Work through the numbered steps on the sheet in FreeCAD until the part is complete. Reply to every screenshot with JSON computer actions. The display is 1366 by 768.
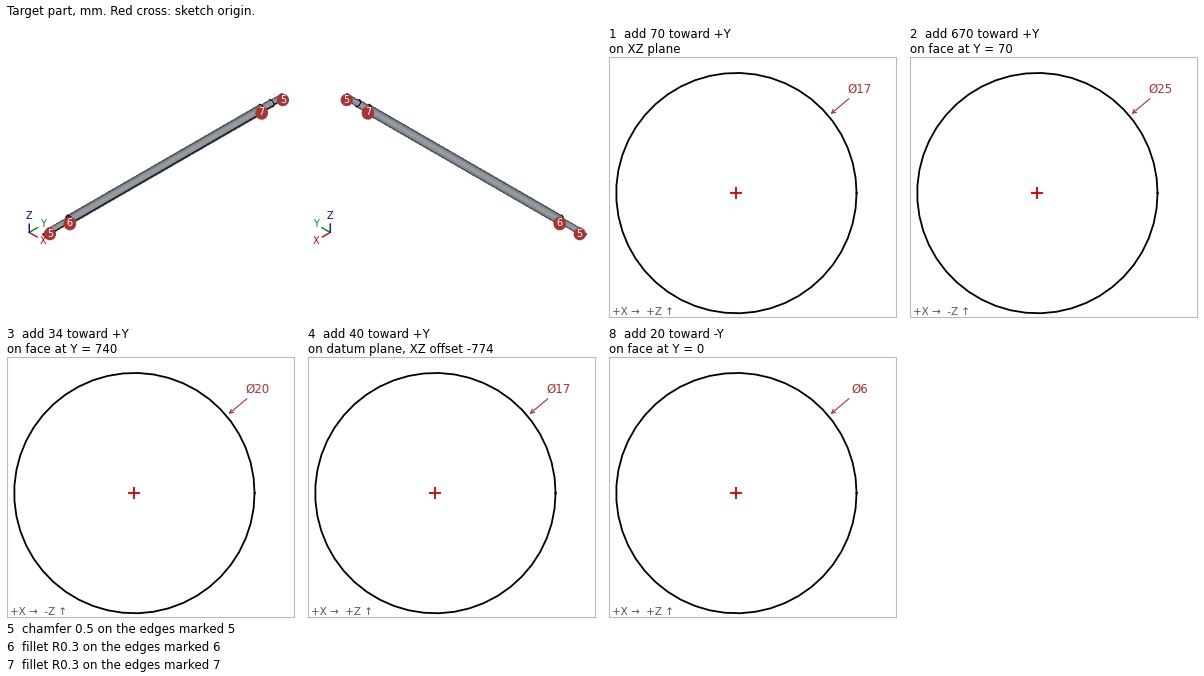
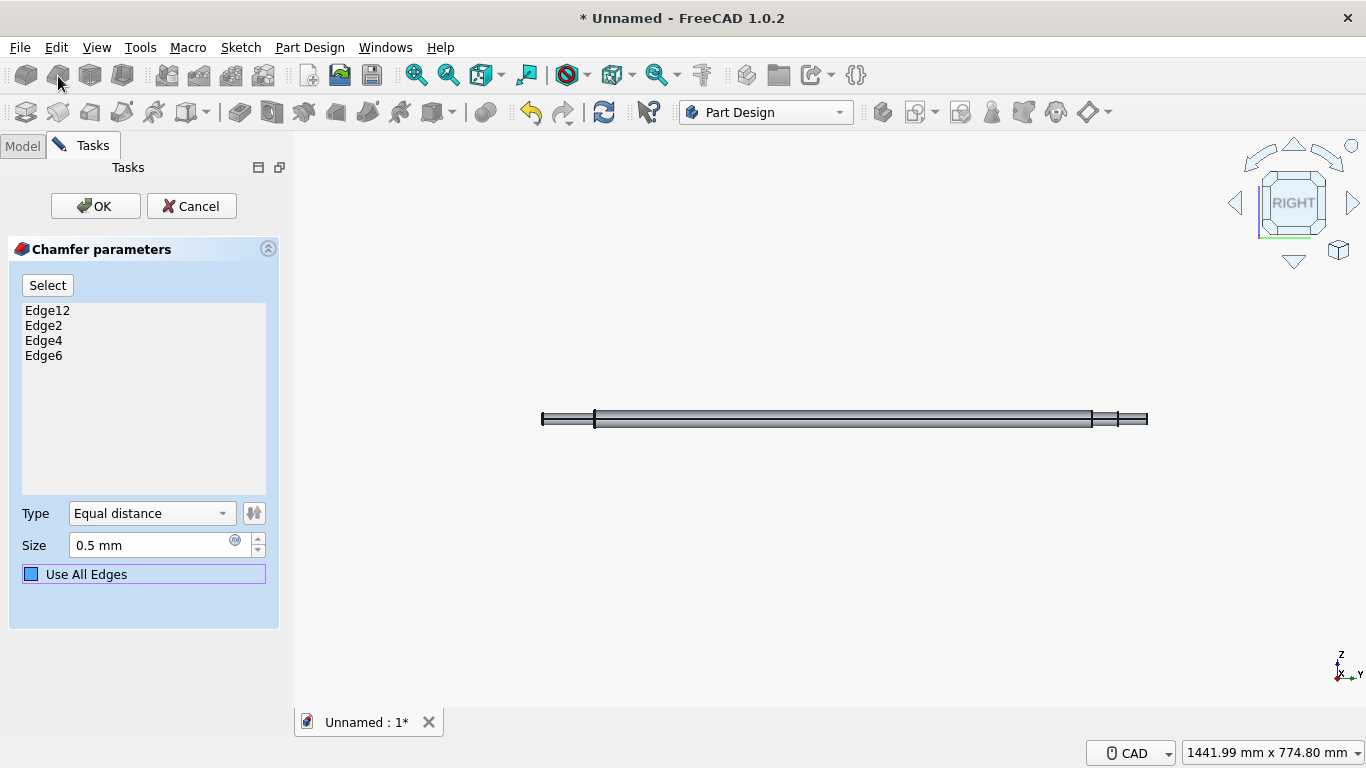
{"action": "left_click", "coordinate": [96, 206]}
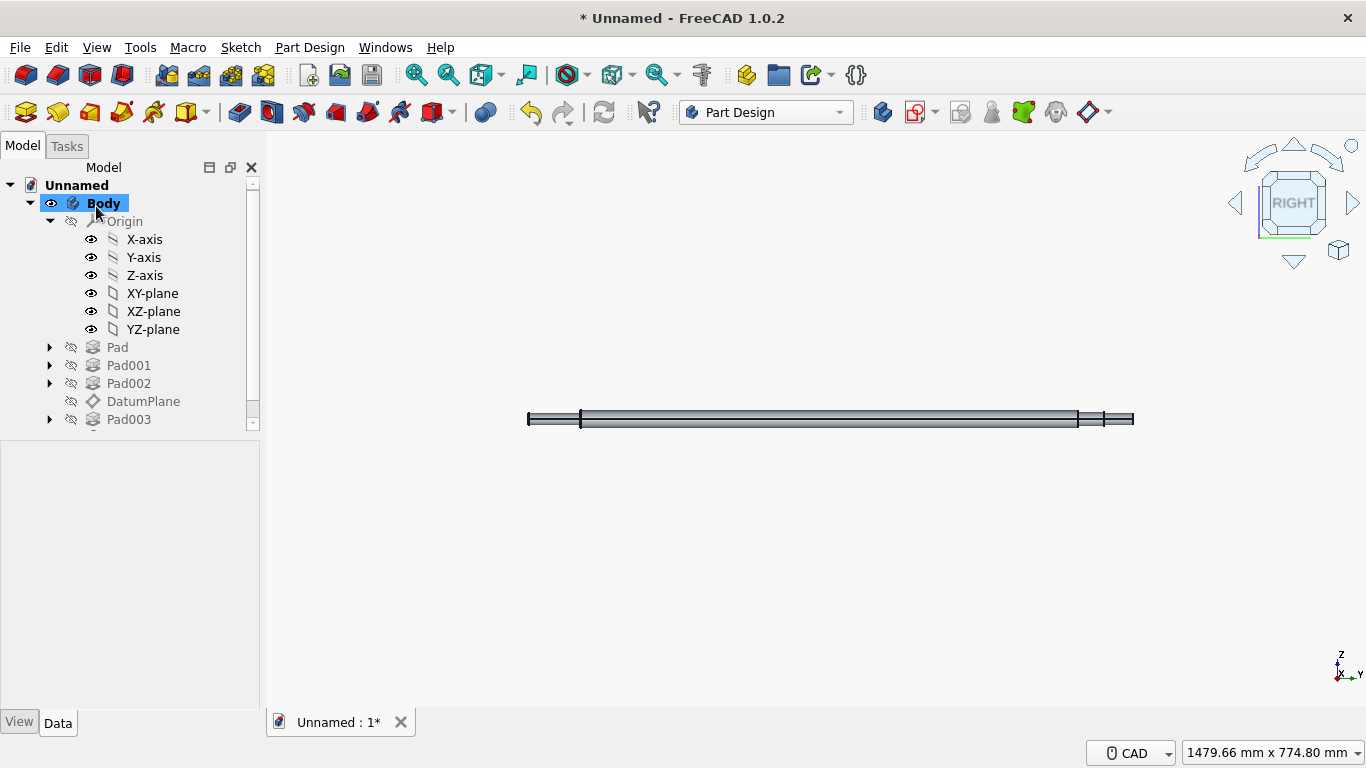
{"action": "key", "text": "0"}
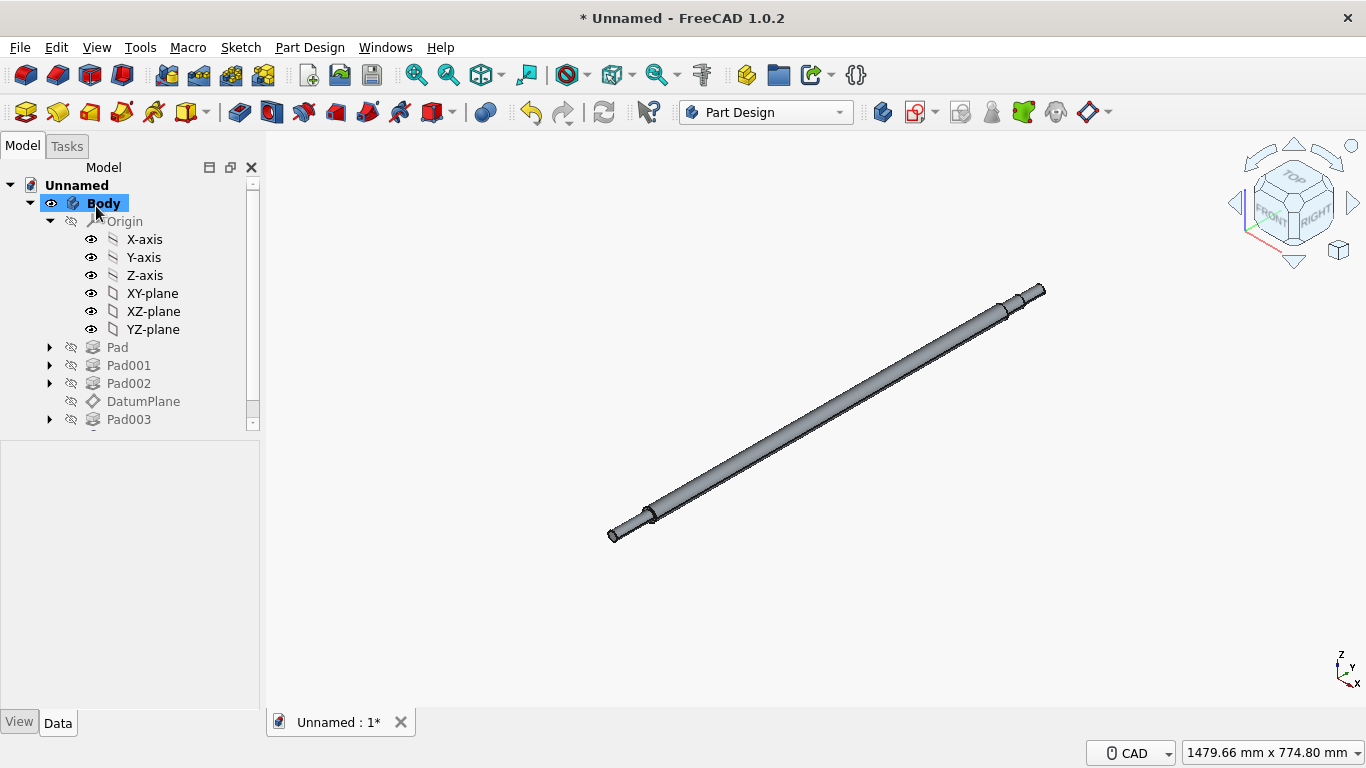
{"action": "key", "text": "2"}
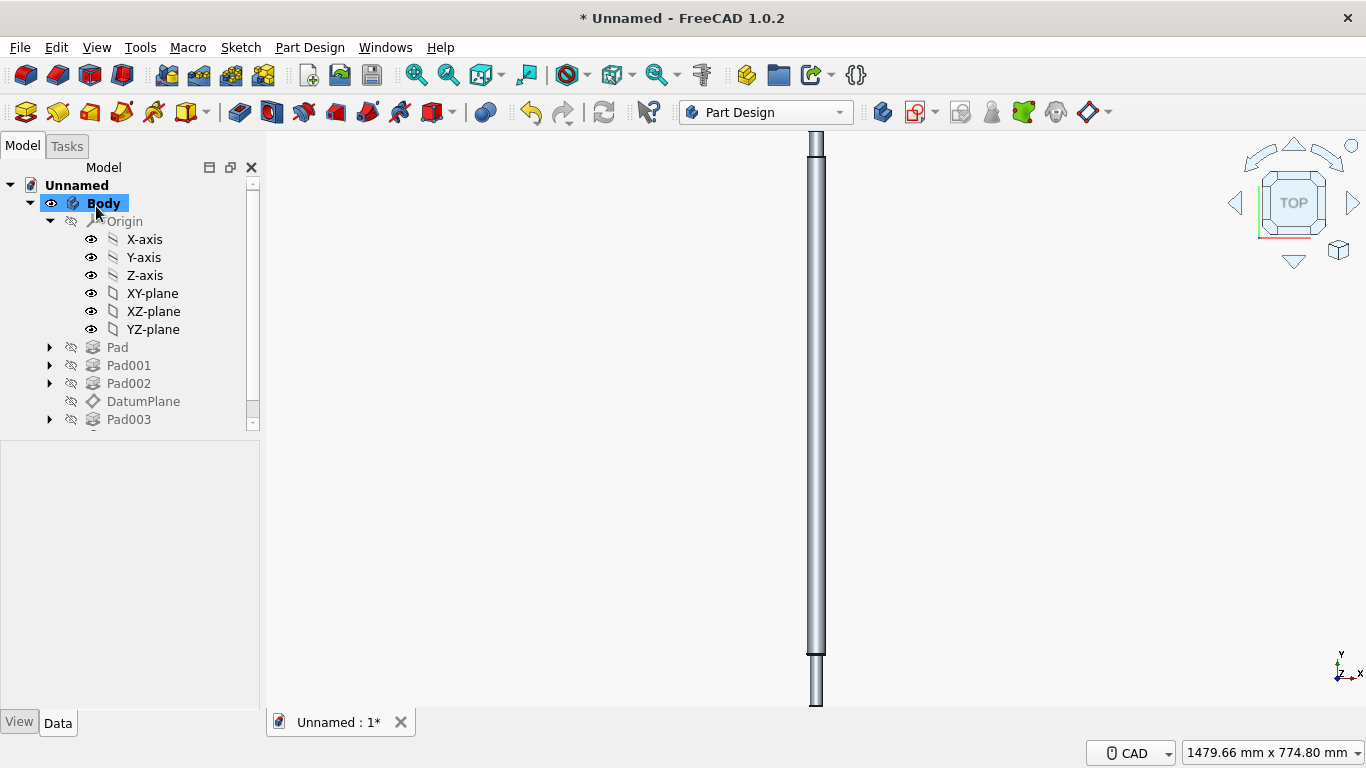
{"action": "left_click", "coordinate": [418, 76]}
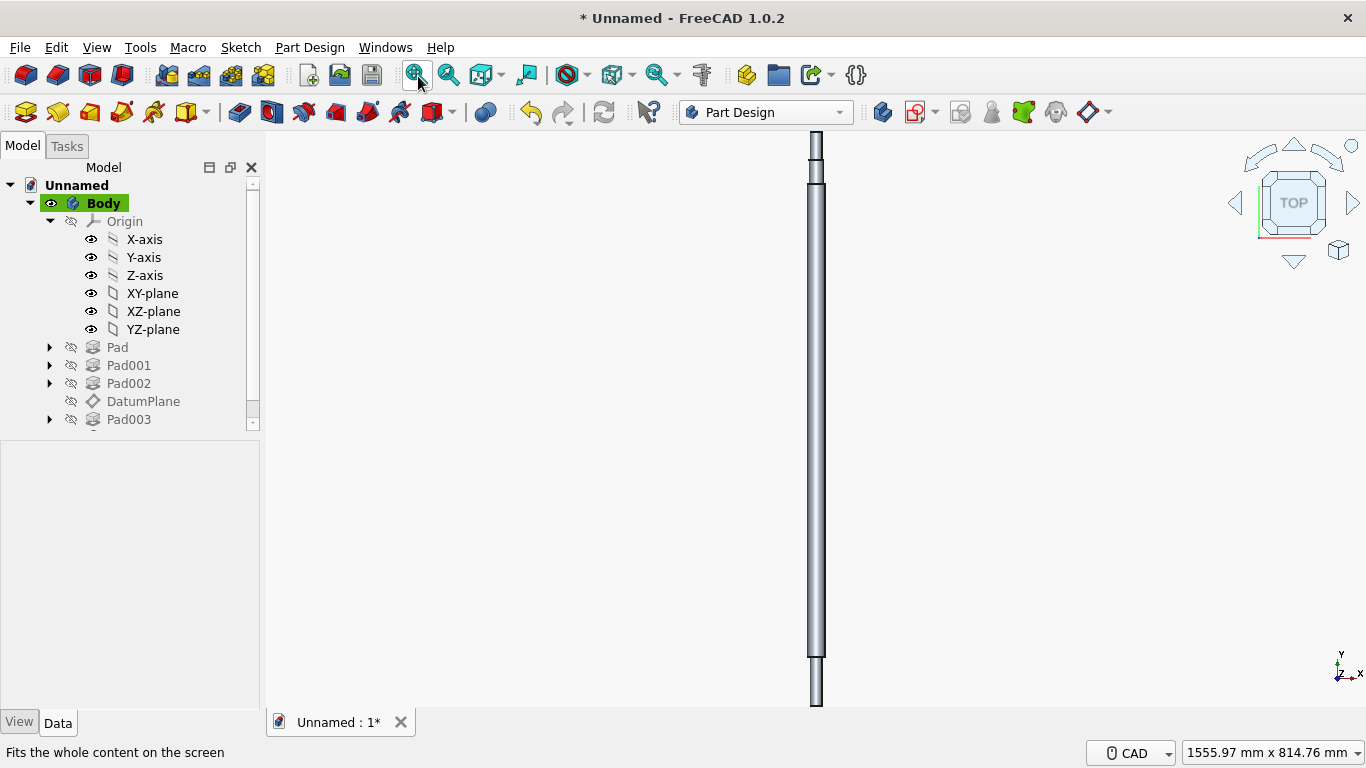
{"action": "key", "text": "1"}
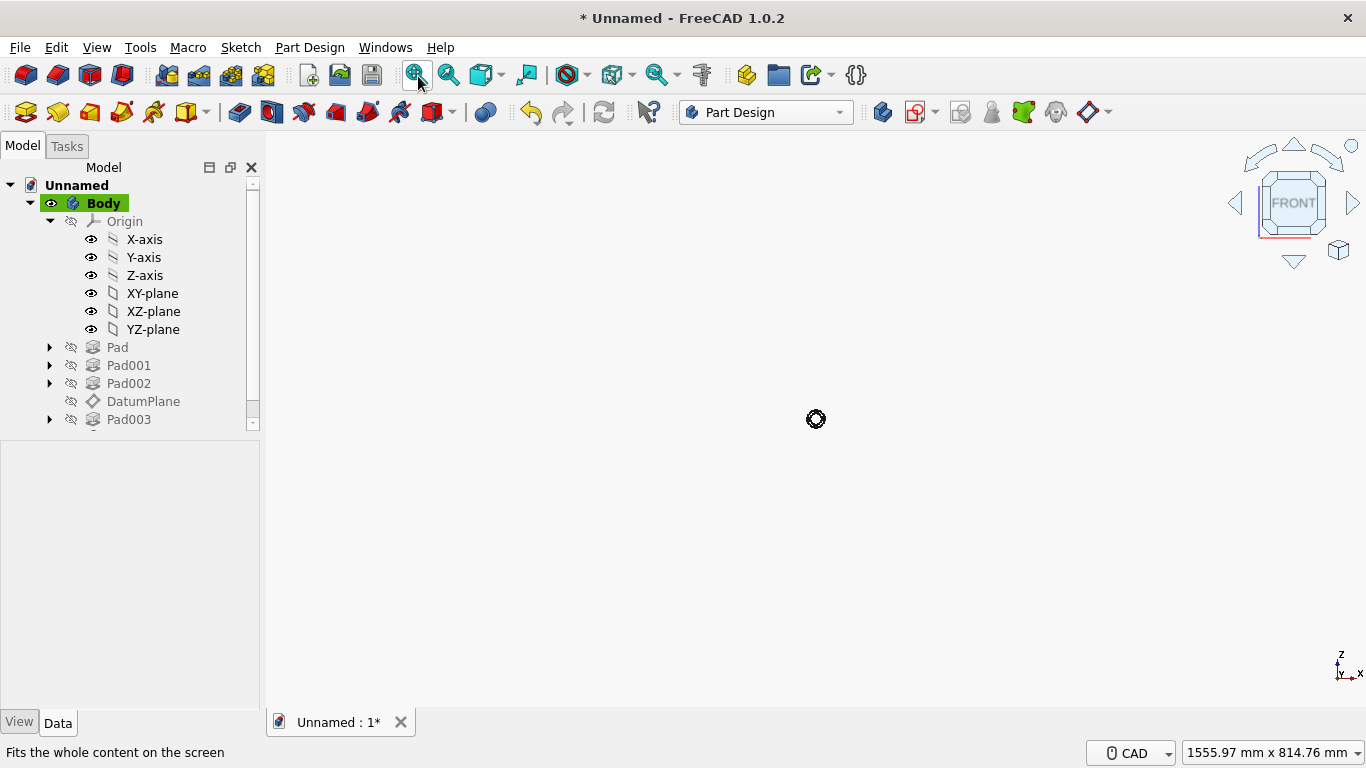
{"action": "key", "text": "v f"}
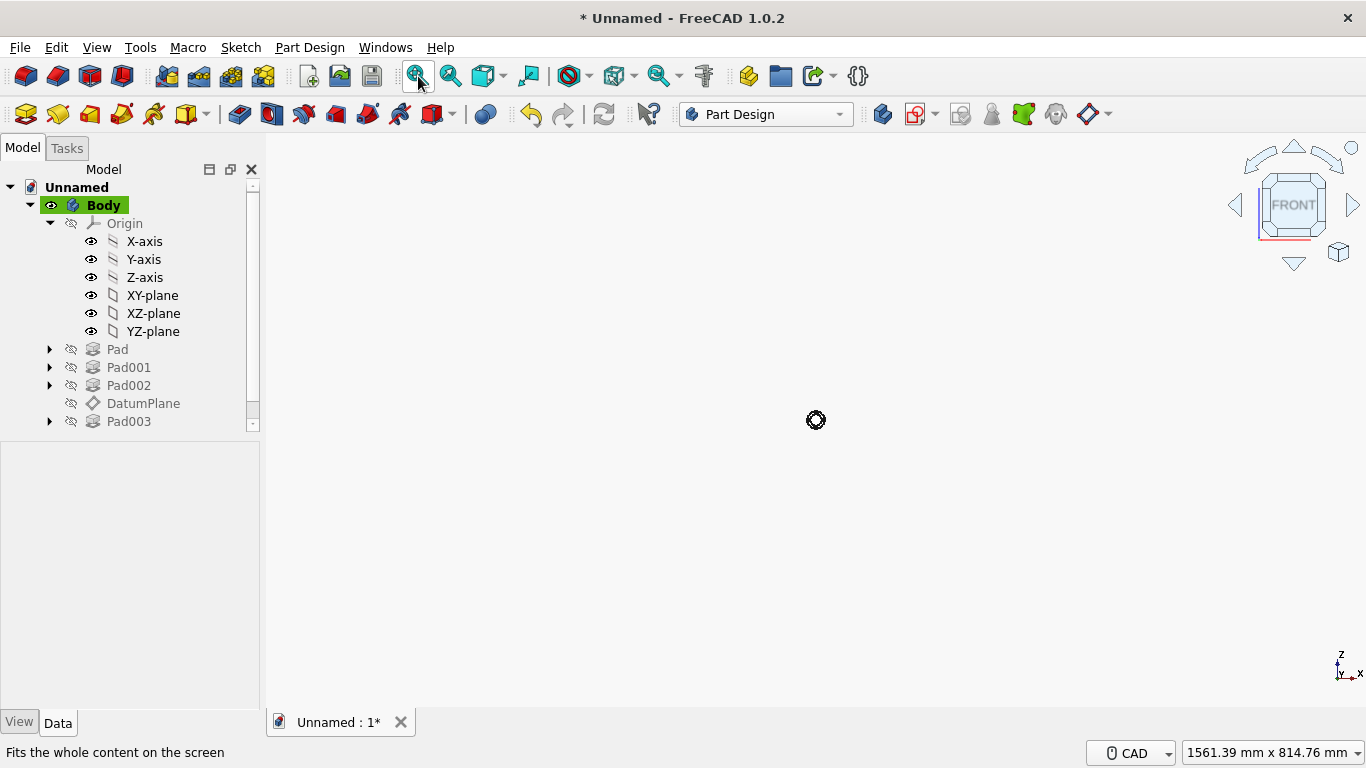
{"action": "key", "text": "3"}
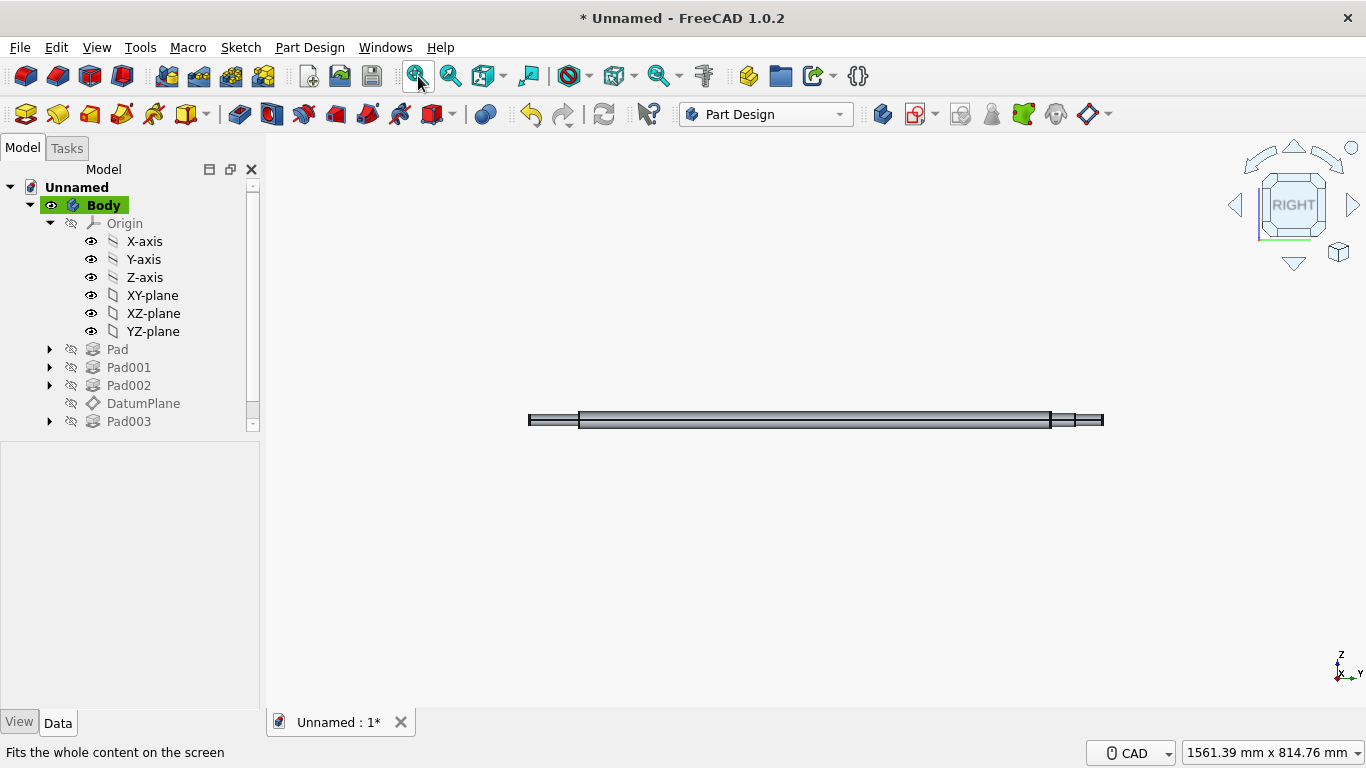
{"action": "key", "text": "5"}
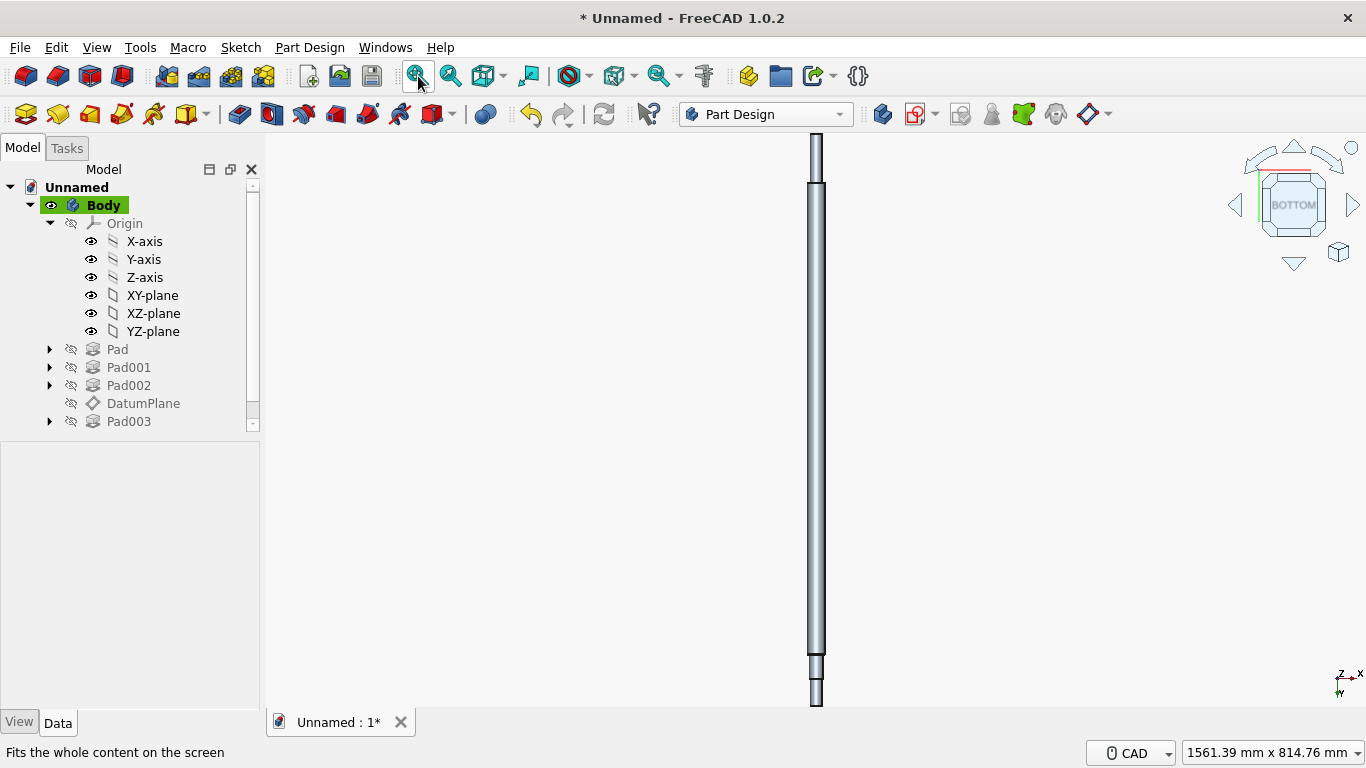
{"action": "key", "text": "v f"}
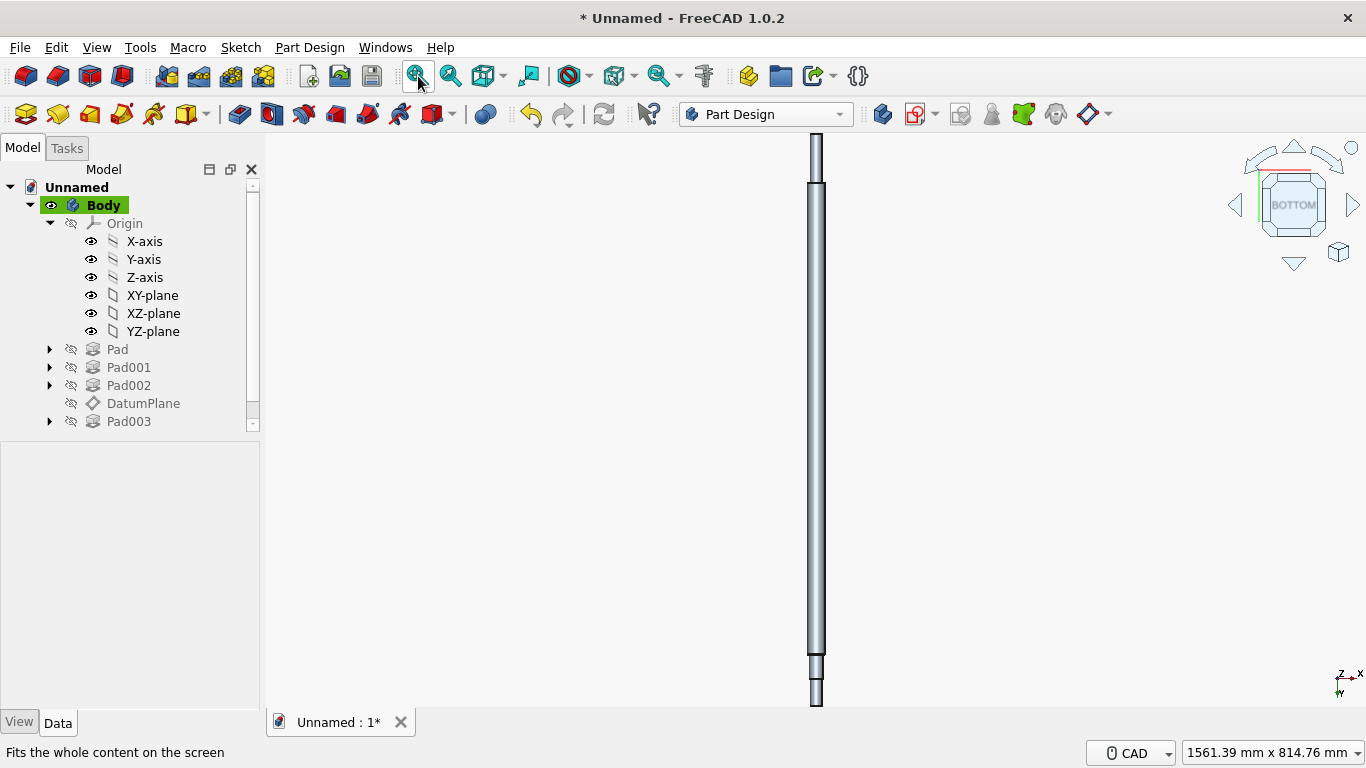
{"action": "key", "text": "4"}